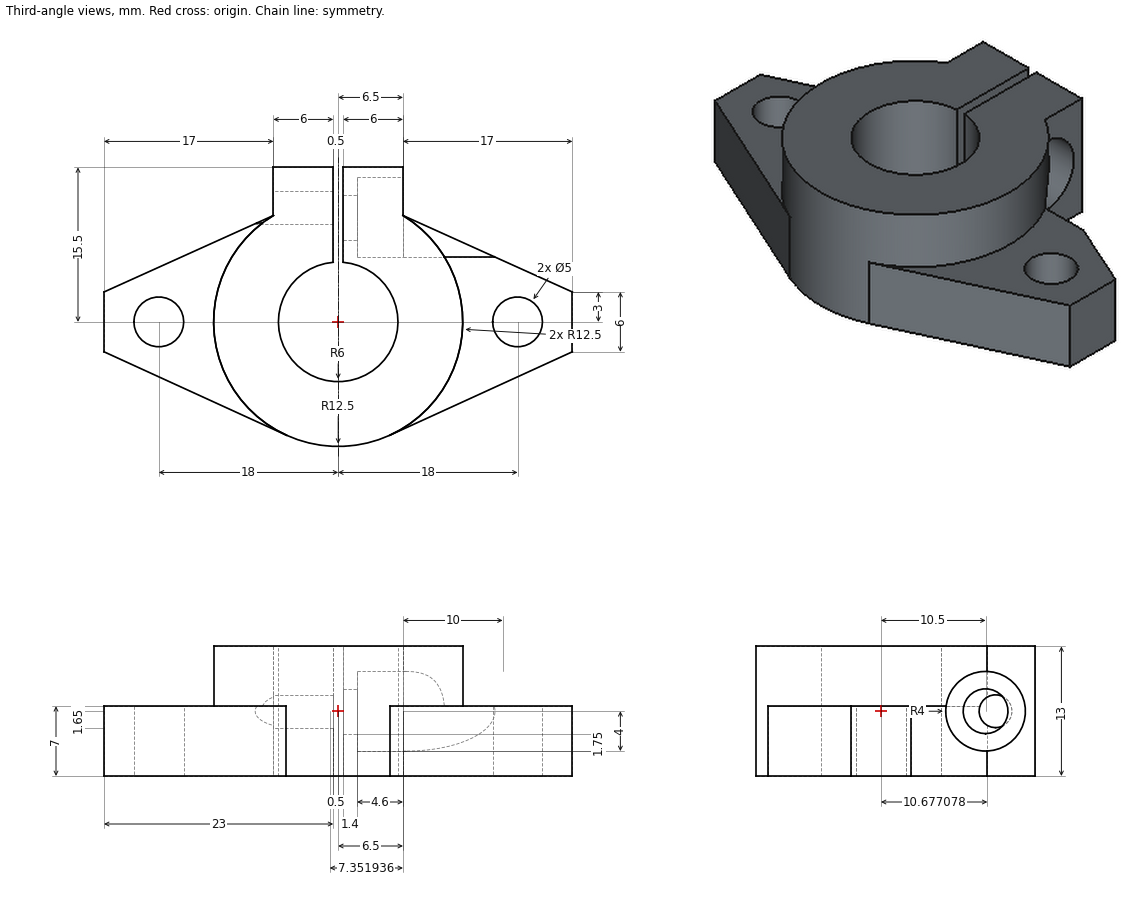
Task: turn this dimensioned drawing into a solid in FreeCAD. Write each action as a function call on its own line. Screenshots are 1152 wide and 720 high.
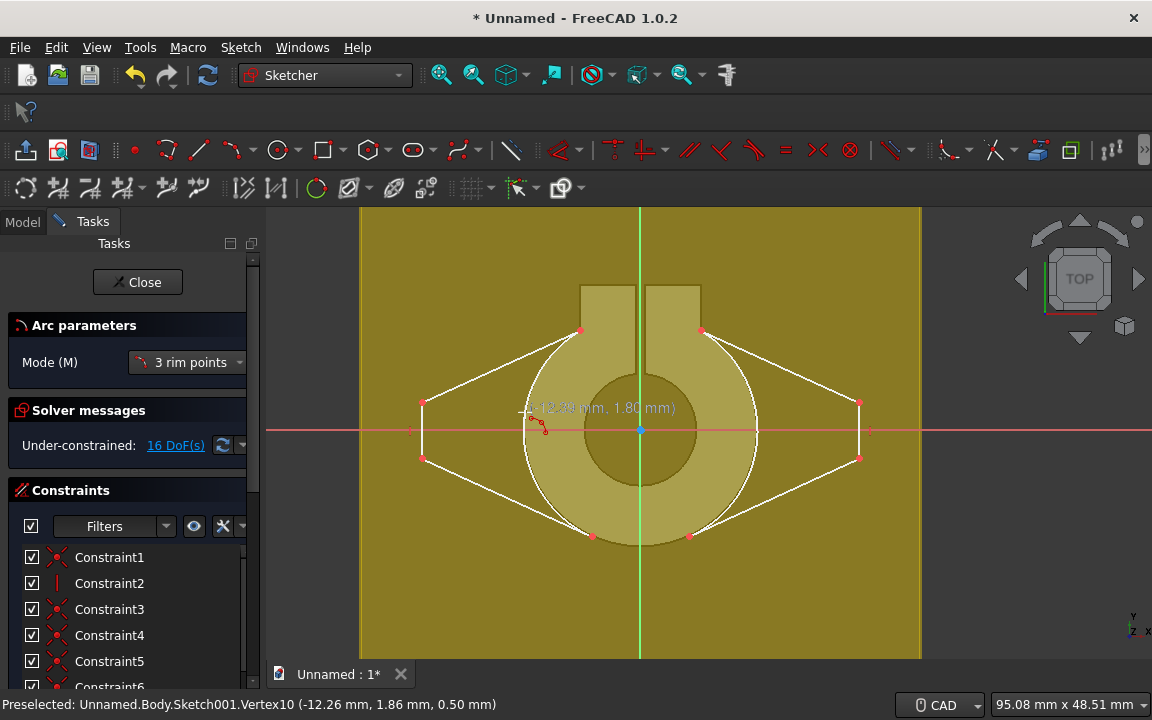
click(278, 150)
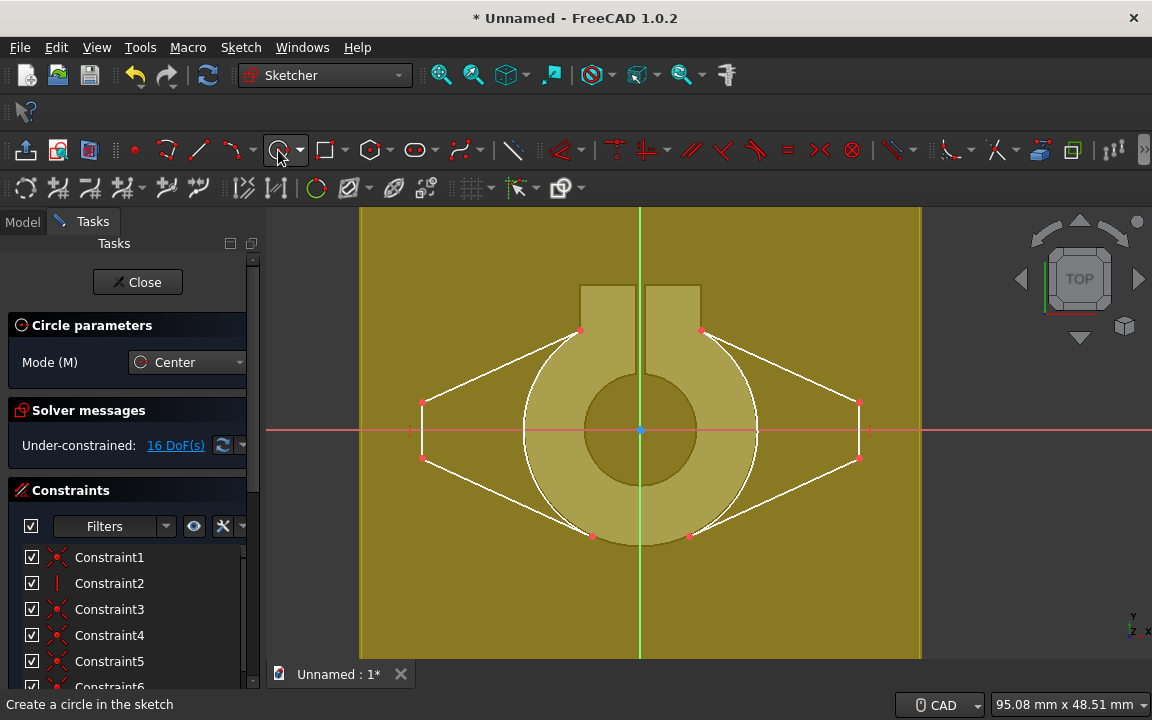
click(808, 430)
click(825, 413)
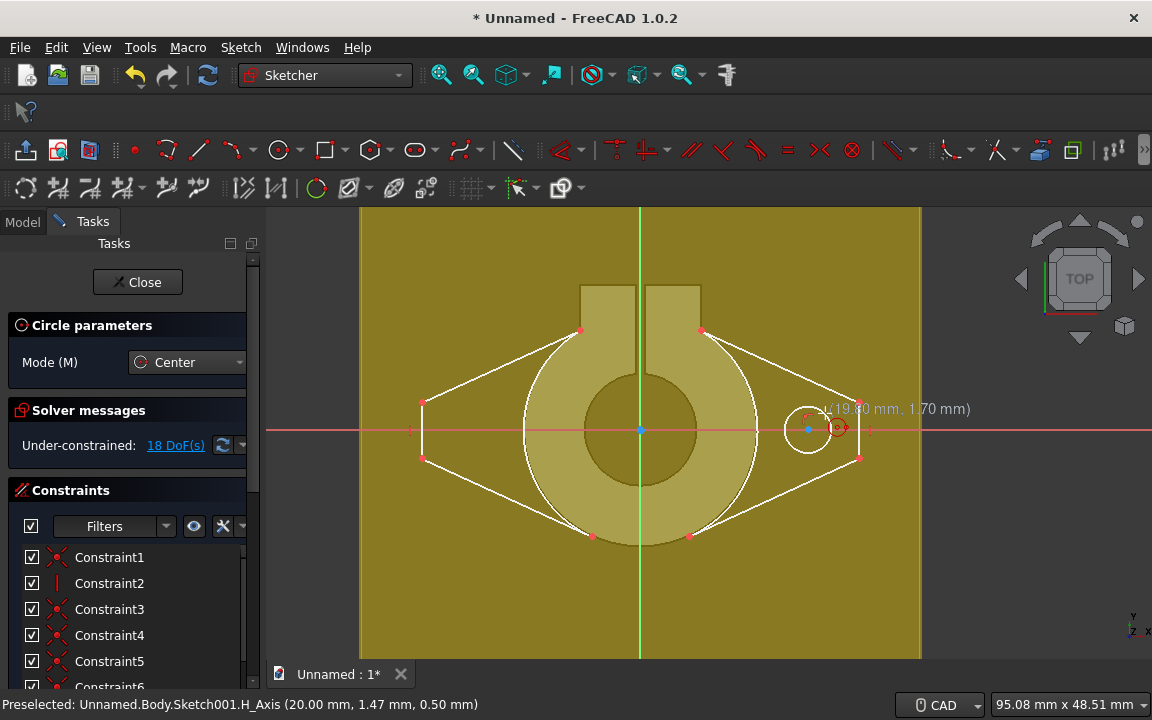
click(473, 430)
click(489, 413)
key(Escape)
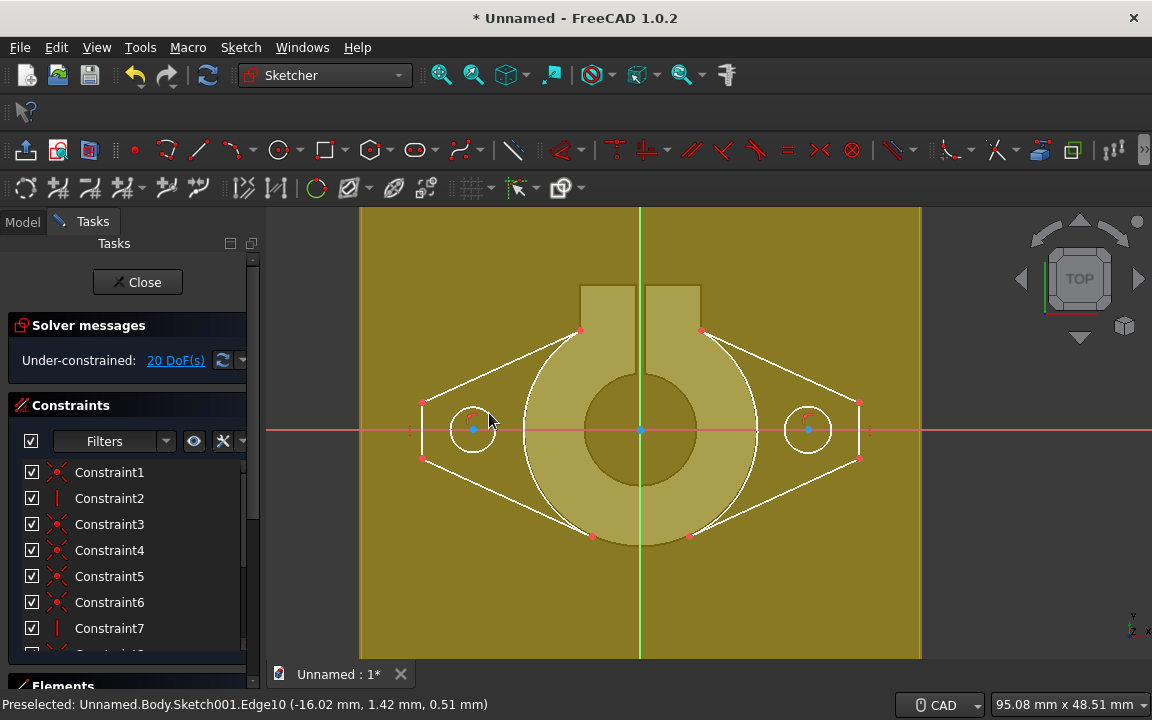
click(808, 482)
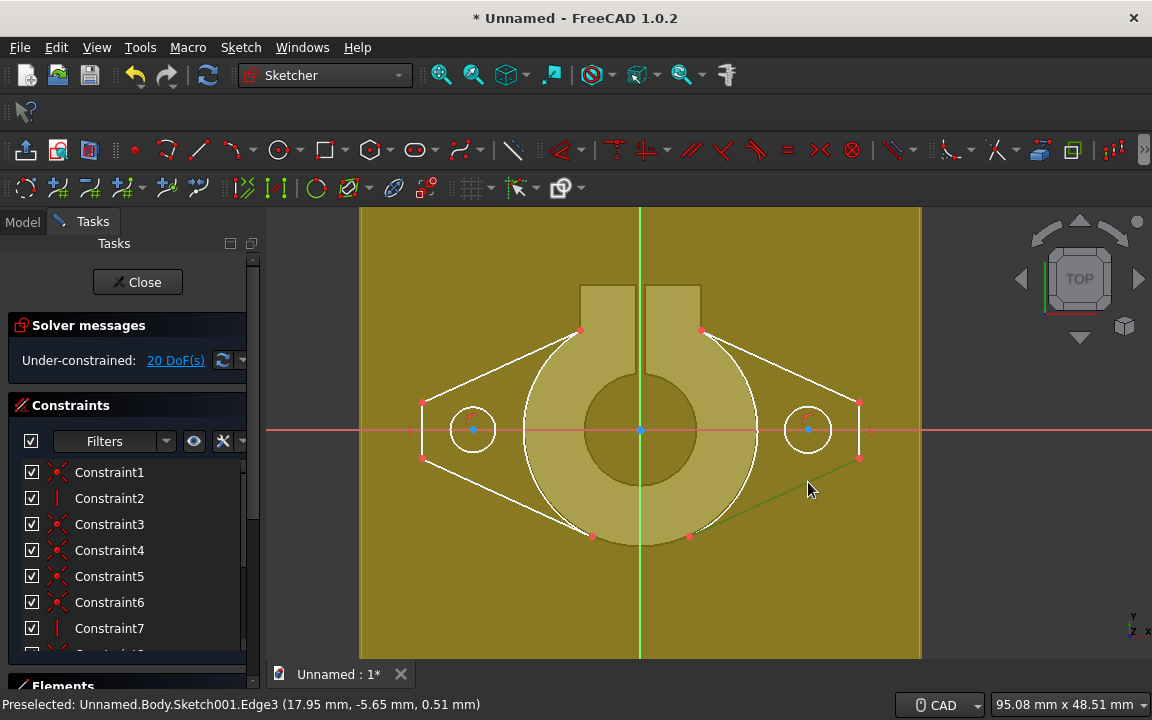
click(744, 486)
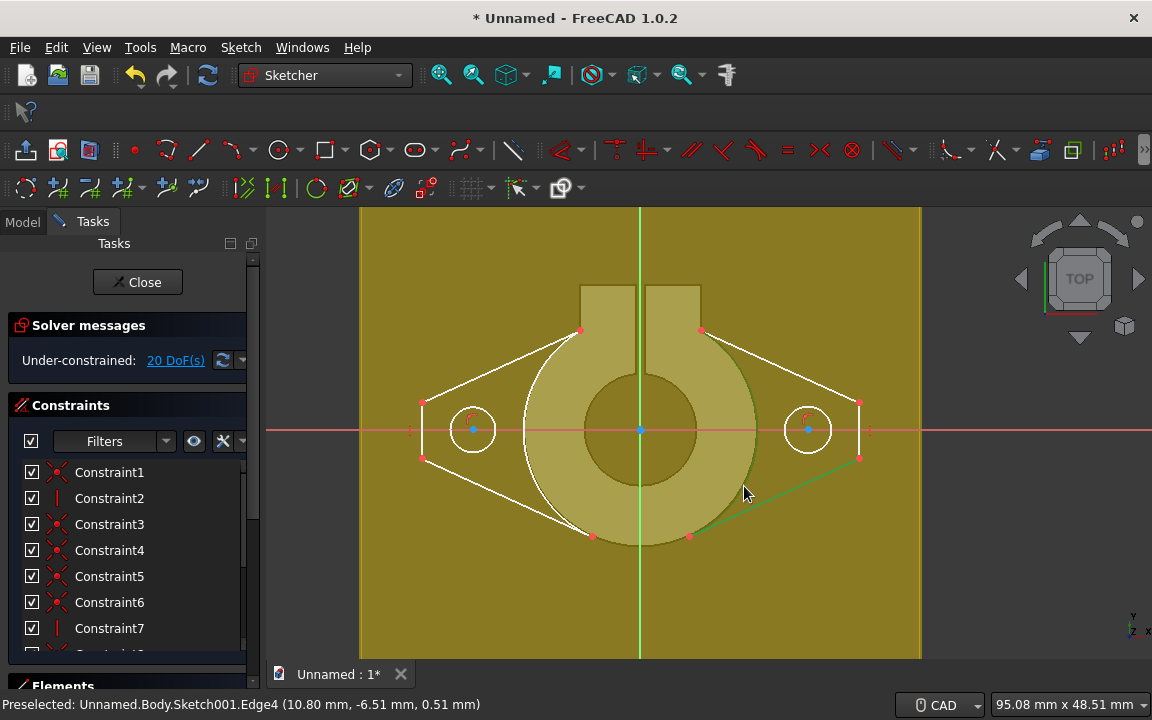
click(756, 150)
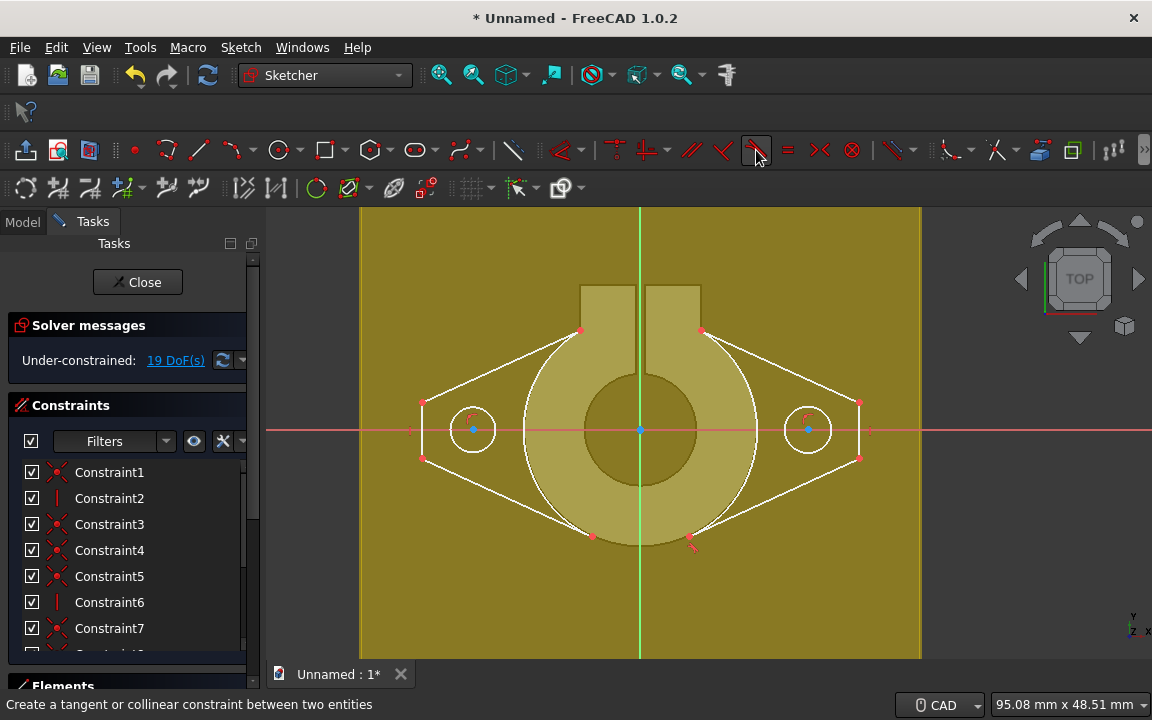
click(541, 514)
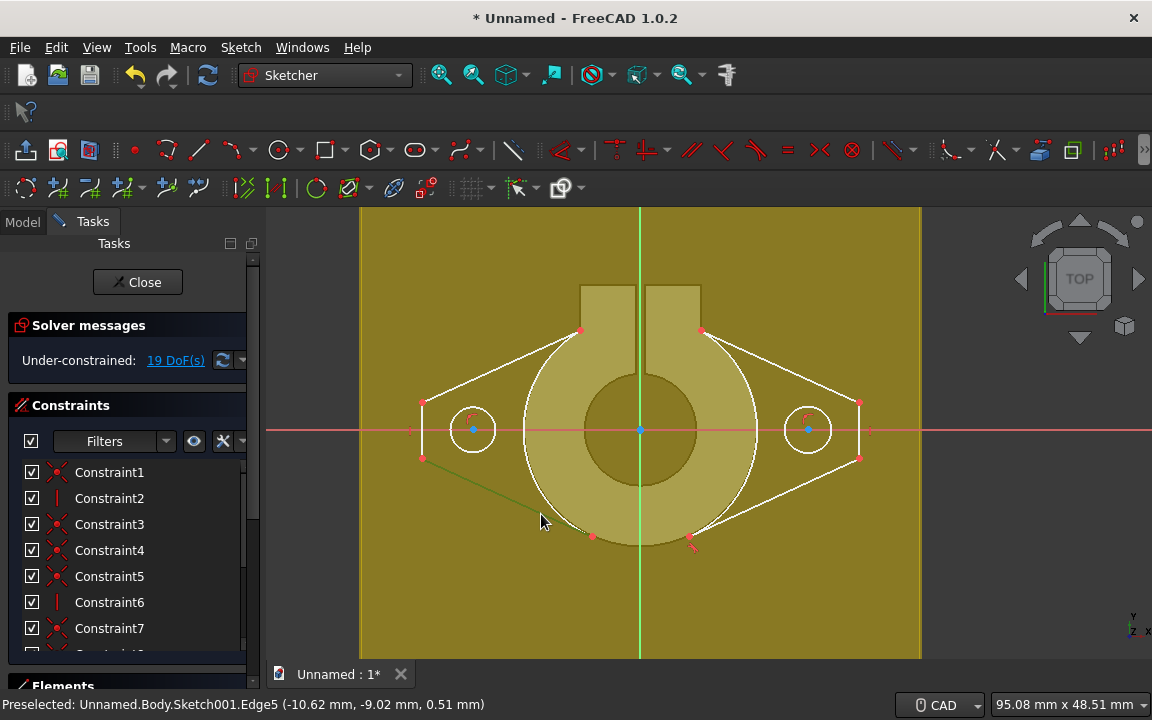
click(532, 388)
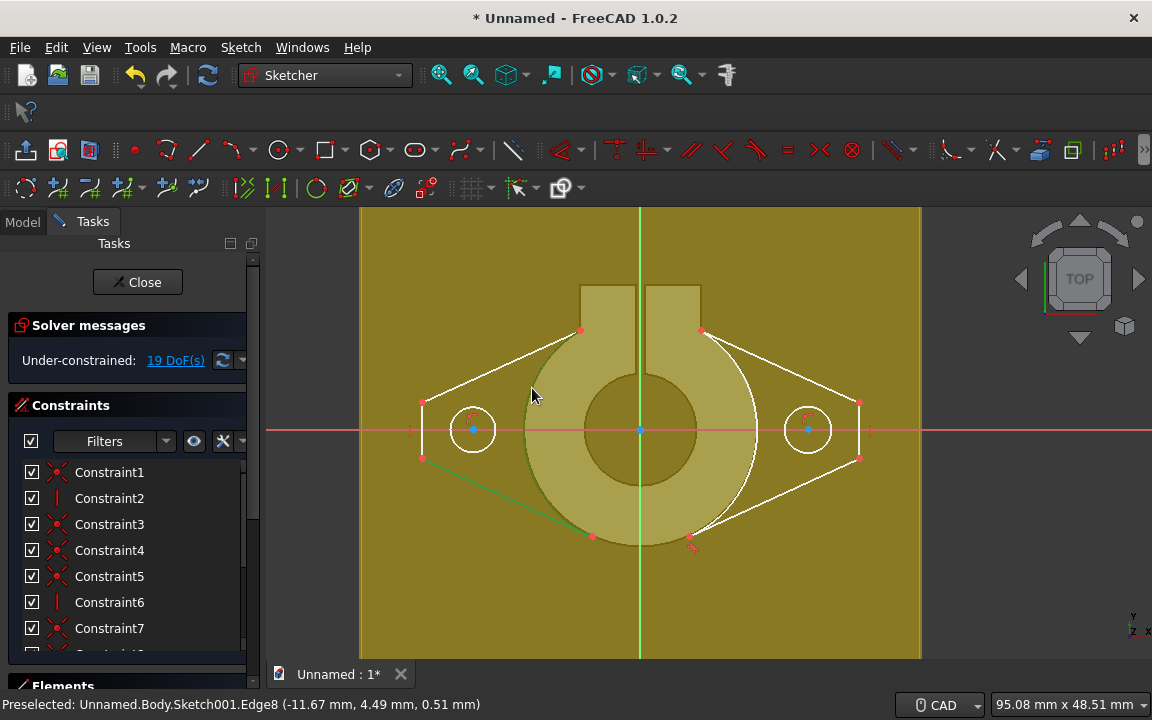
click(756, 150)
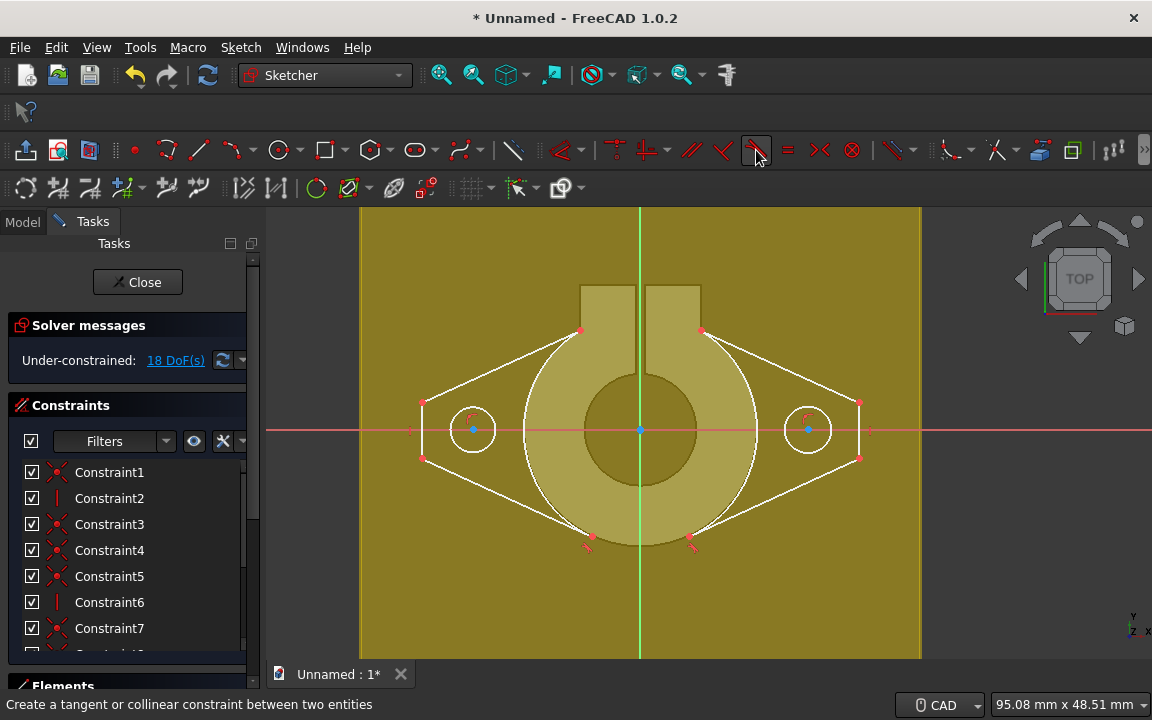
click(743, 486)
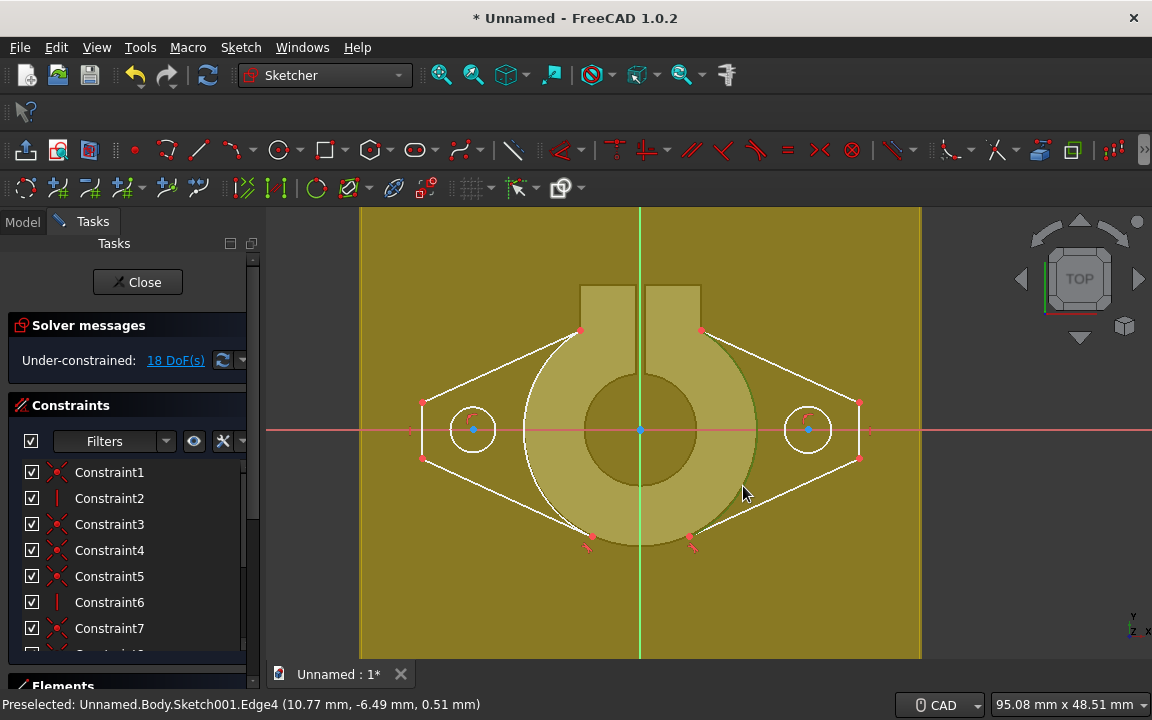
click(532, 388)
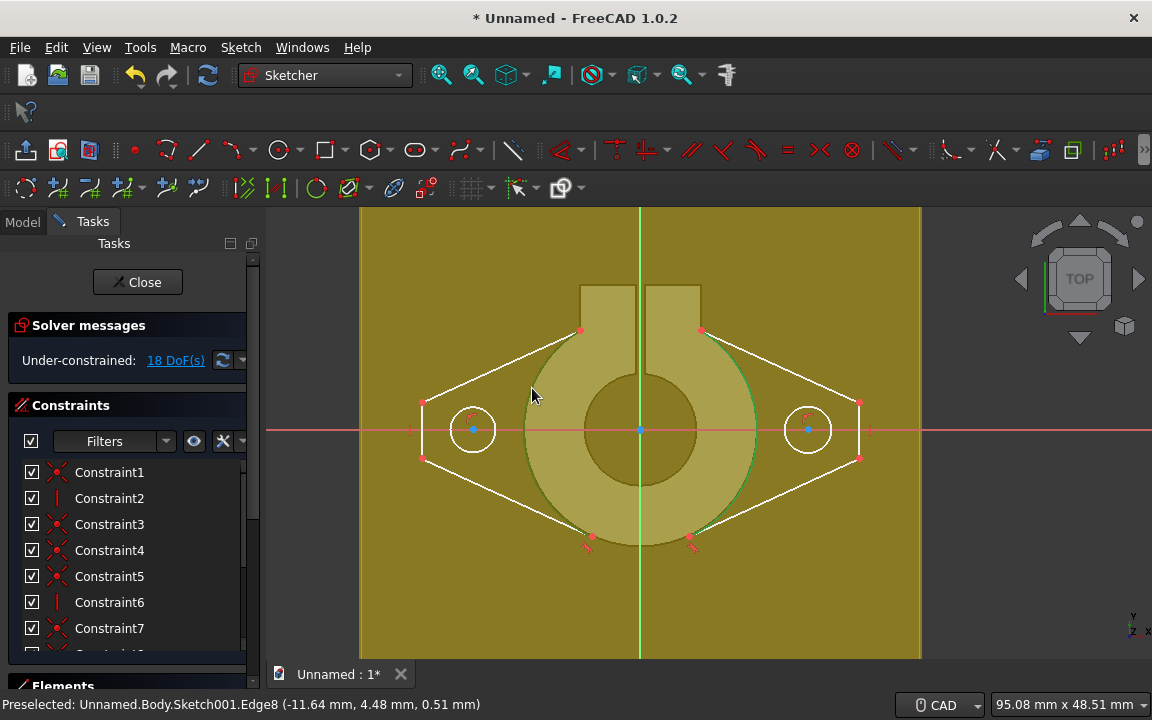
click(616, 150)